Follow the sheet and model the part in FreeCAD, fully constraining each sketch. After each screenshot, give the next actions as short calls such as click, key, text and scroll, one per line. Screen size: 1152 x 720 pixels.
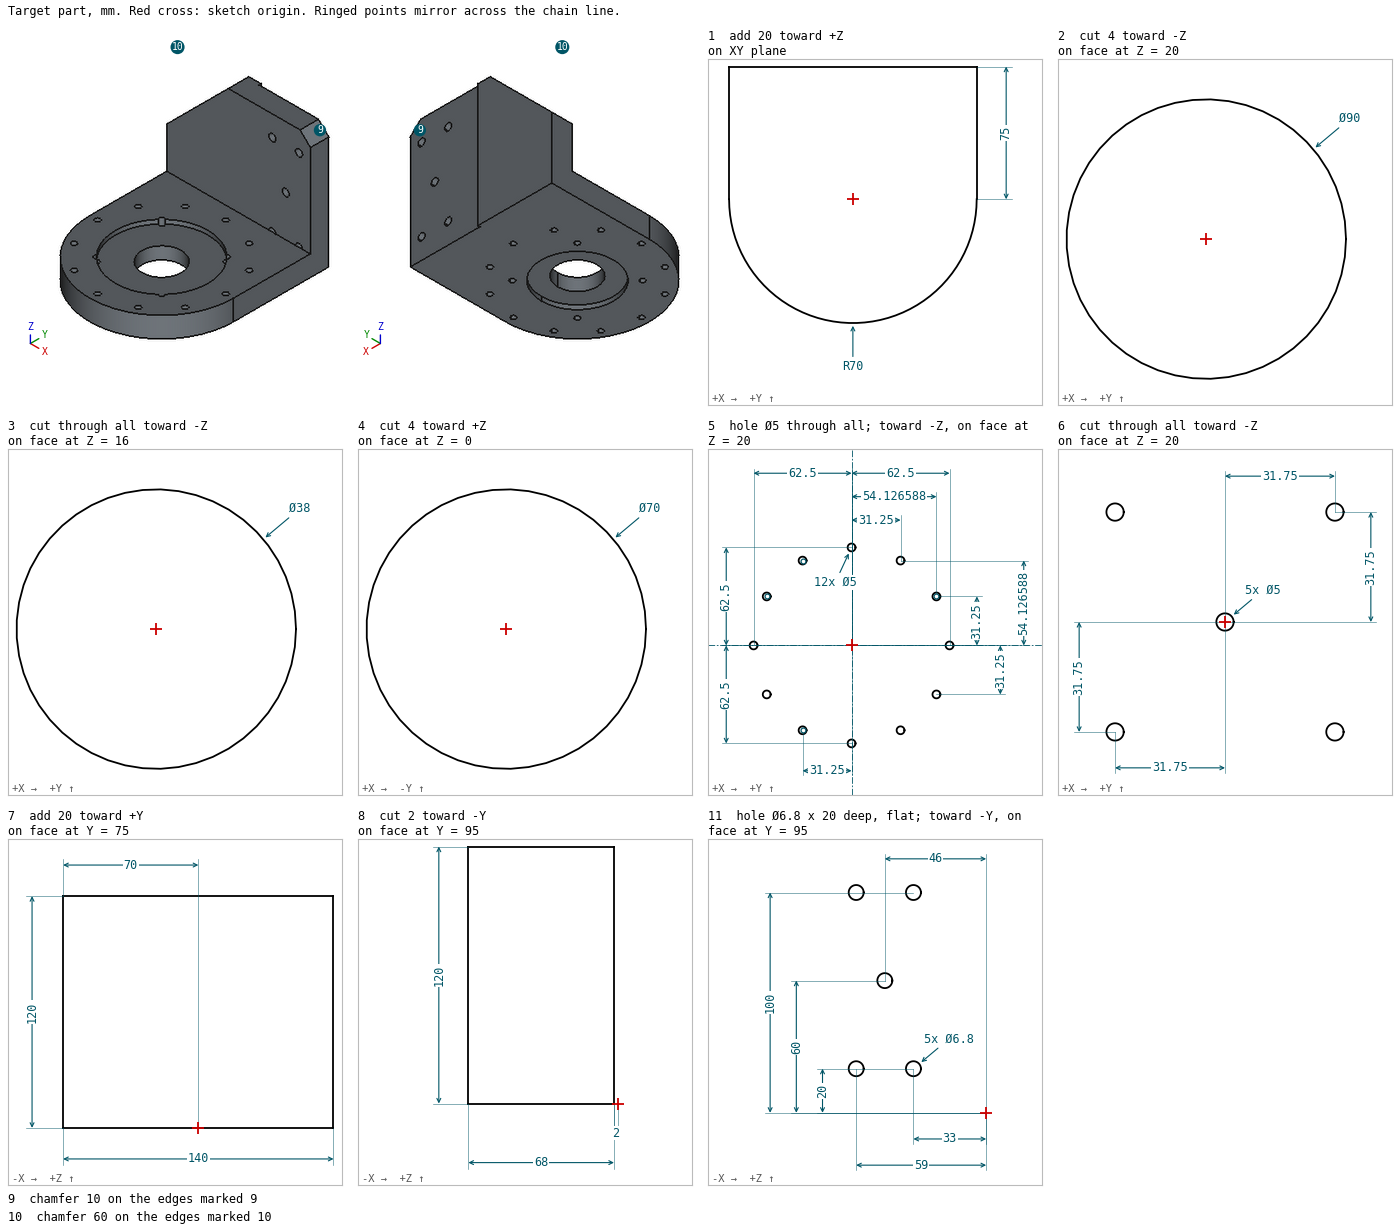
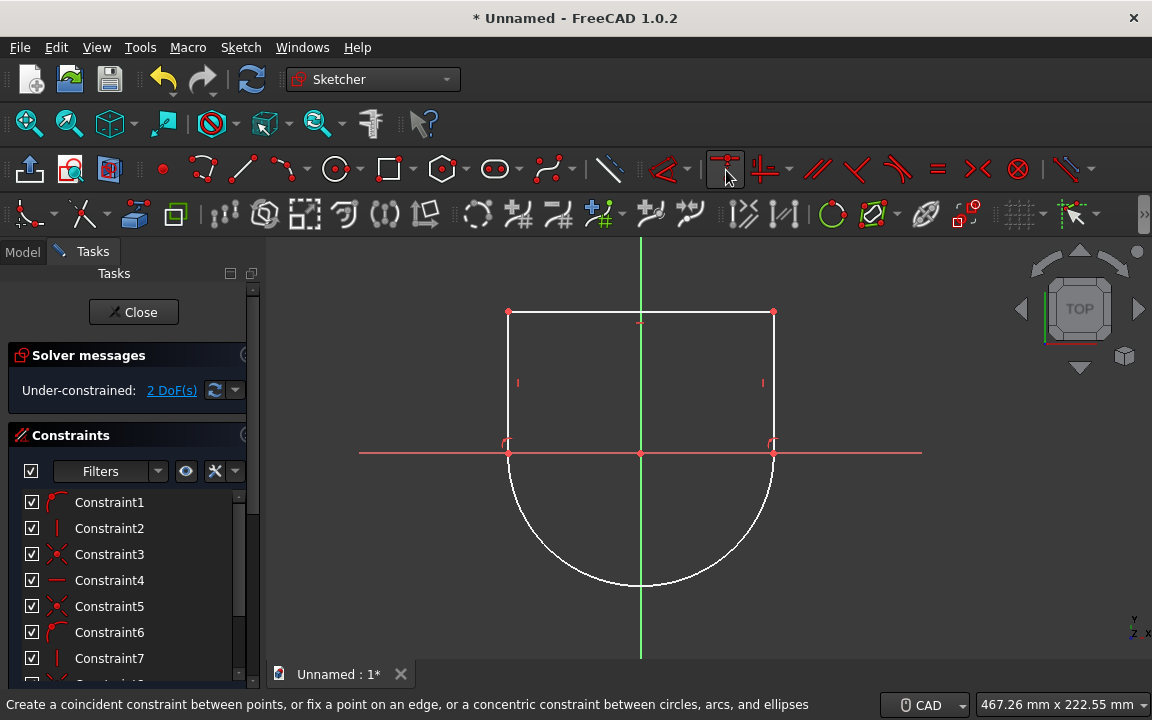
click(664, 170)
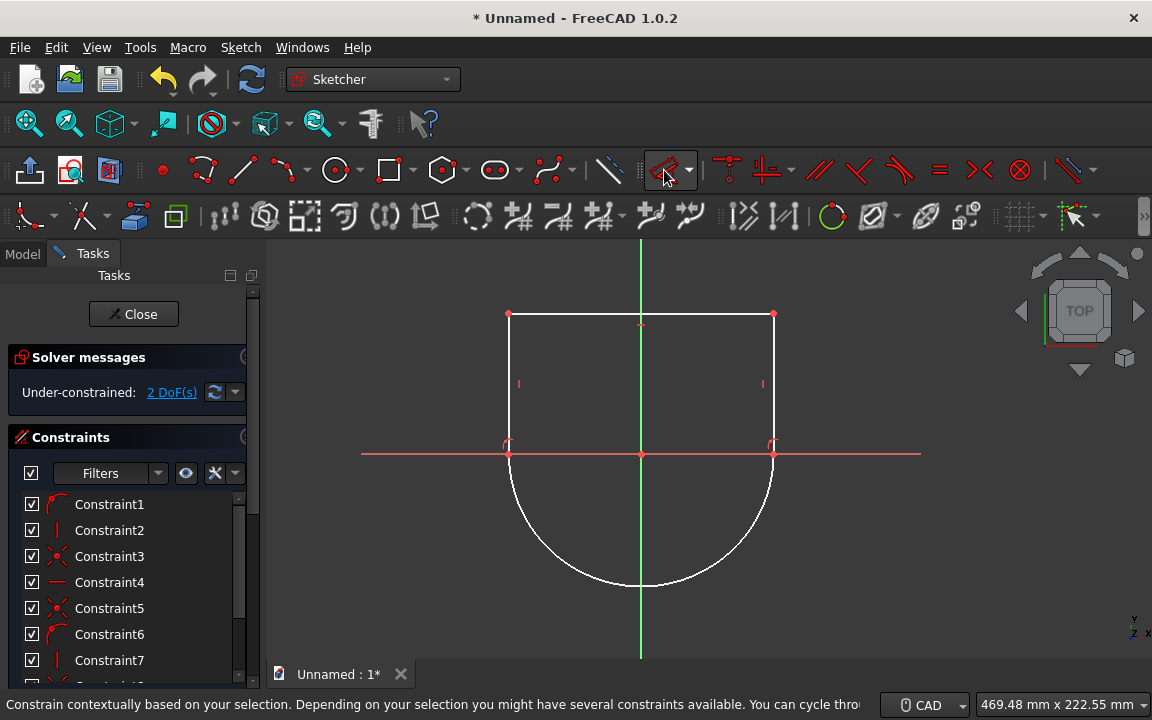
click(563, 561)
click(544, 587)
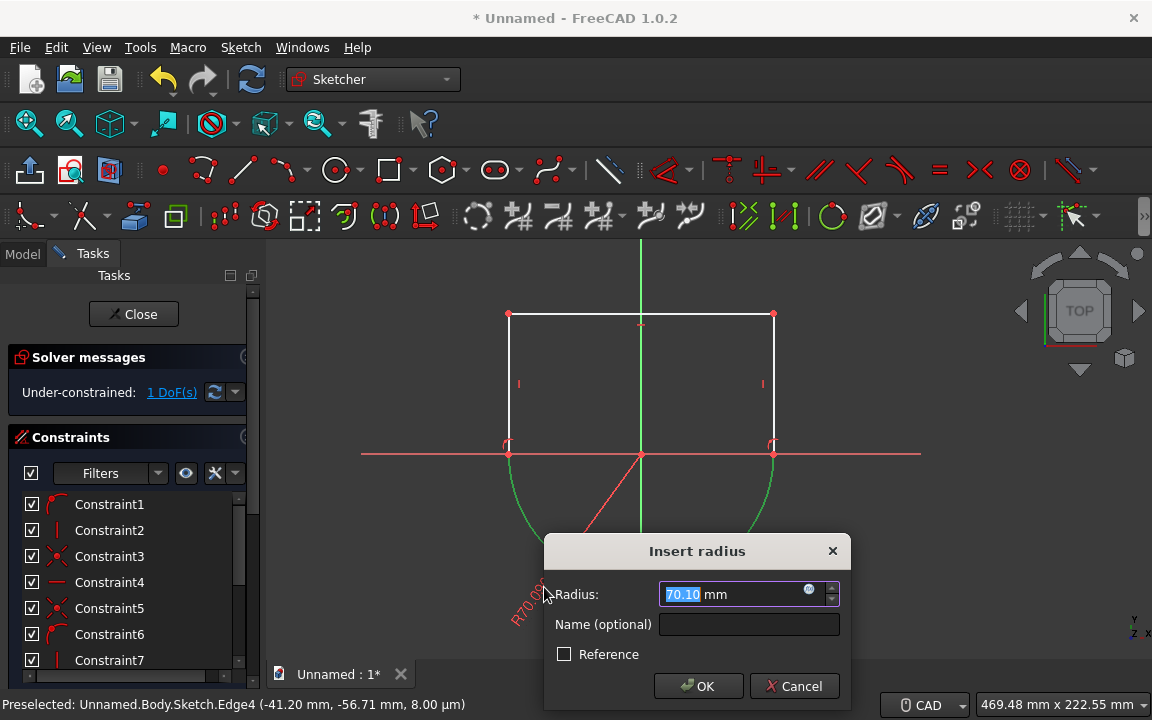
text(70)
key(Return)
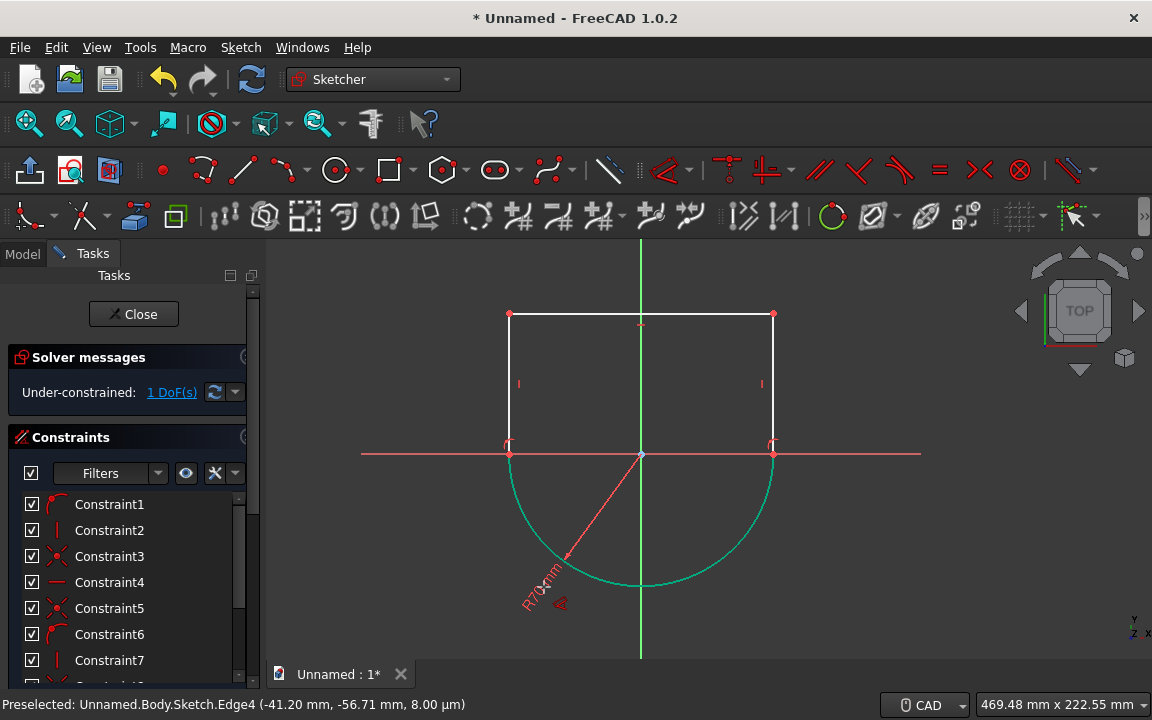
click(773, 412)
click(807, 384)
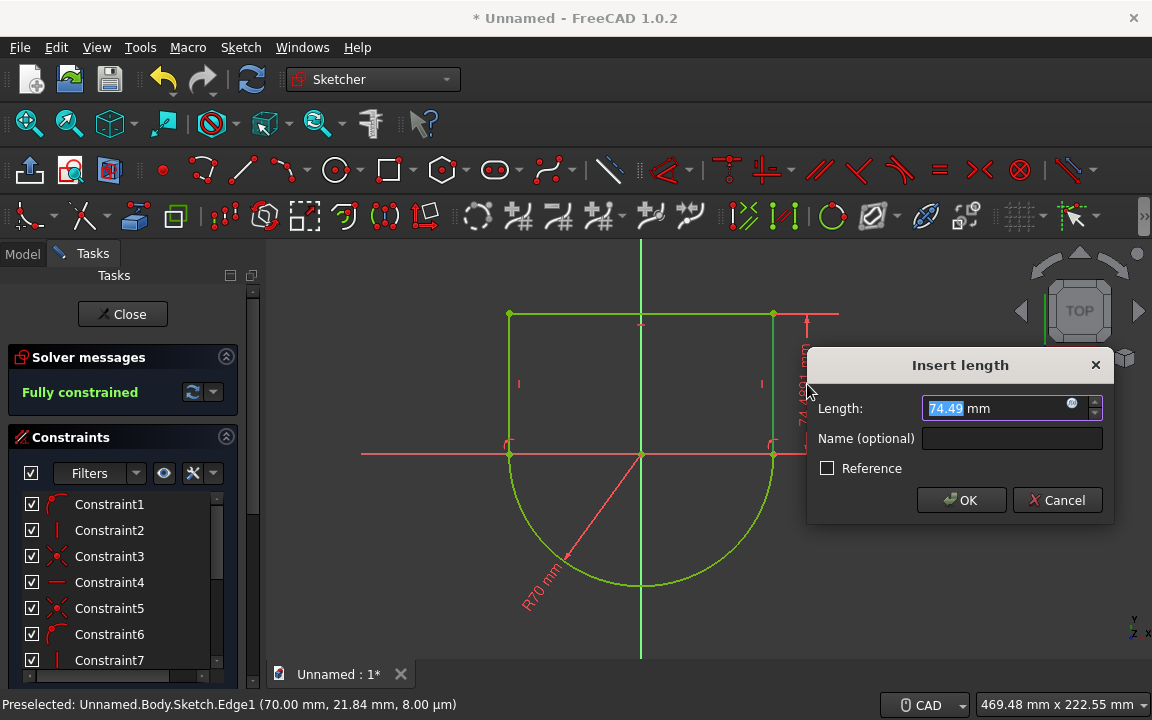
text(75)
key(Return)
key(Escape)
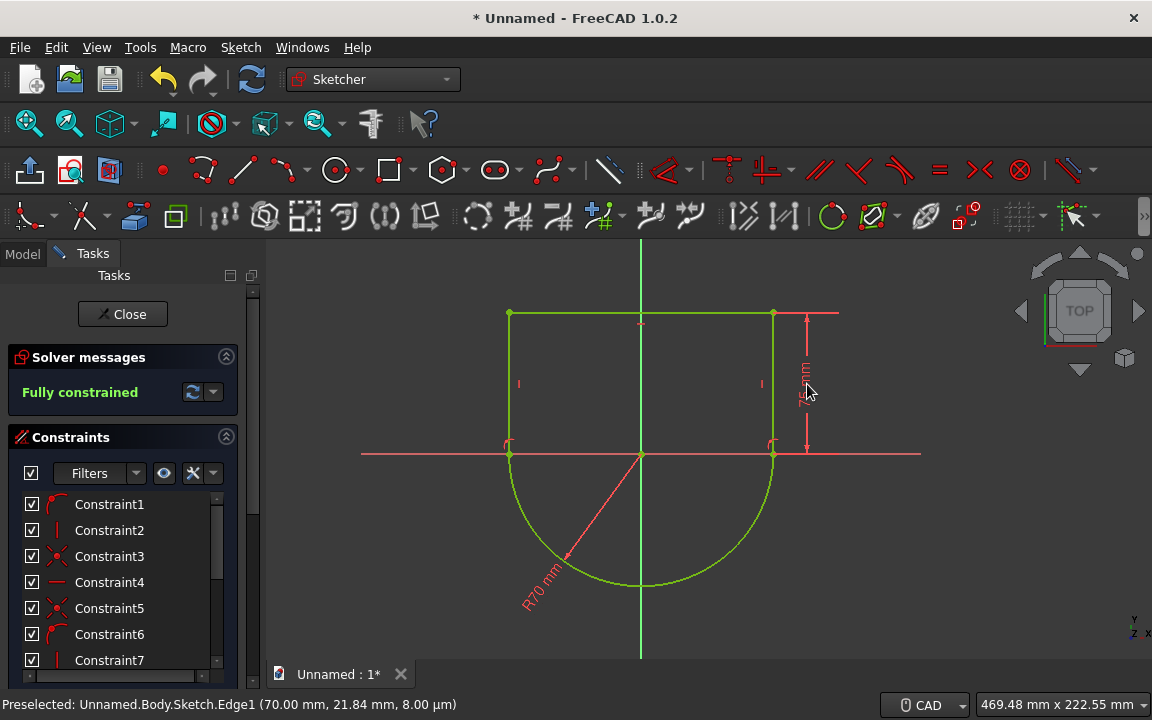
click(123, 314)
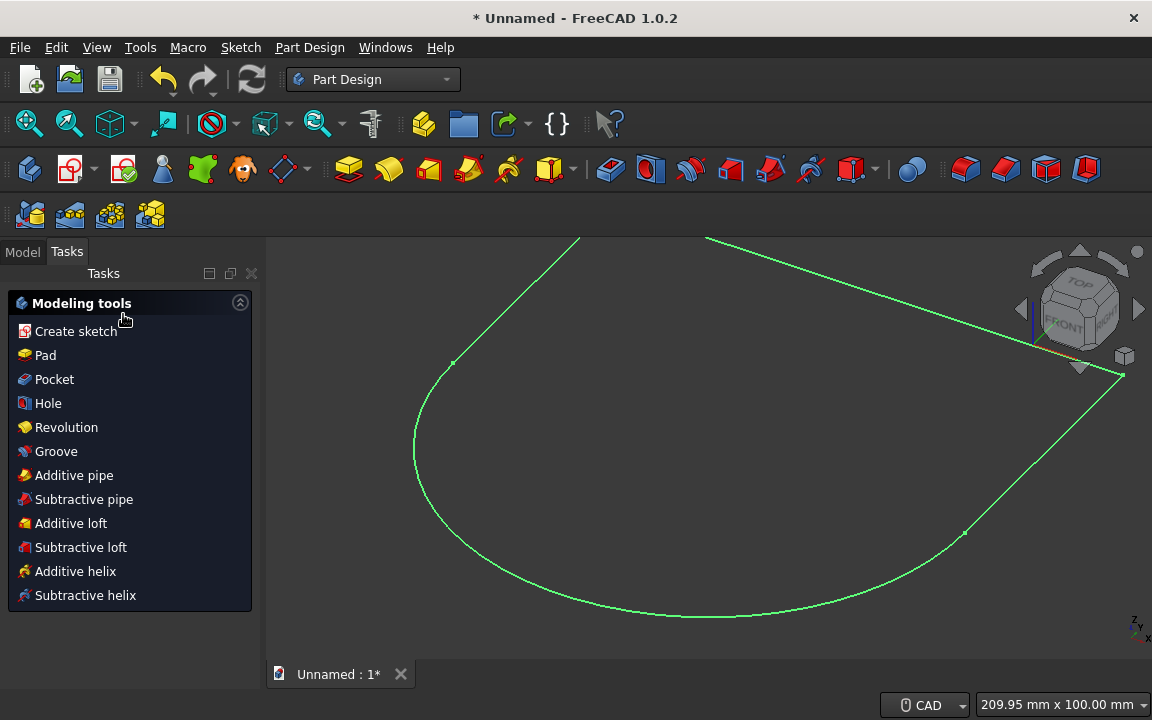
click(350, 170)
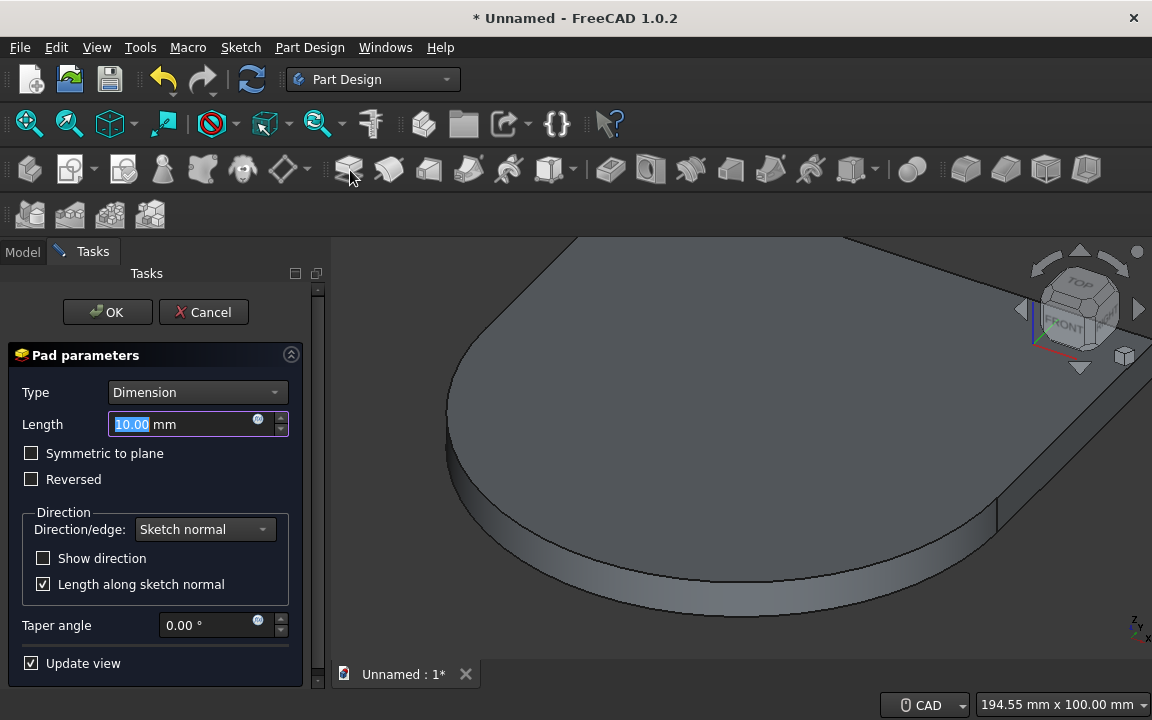
text(20)
key(Tab)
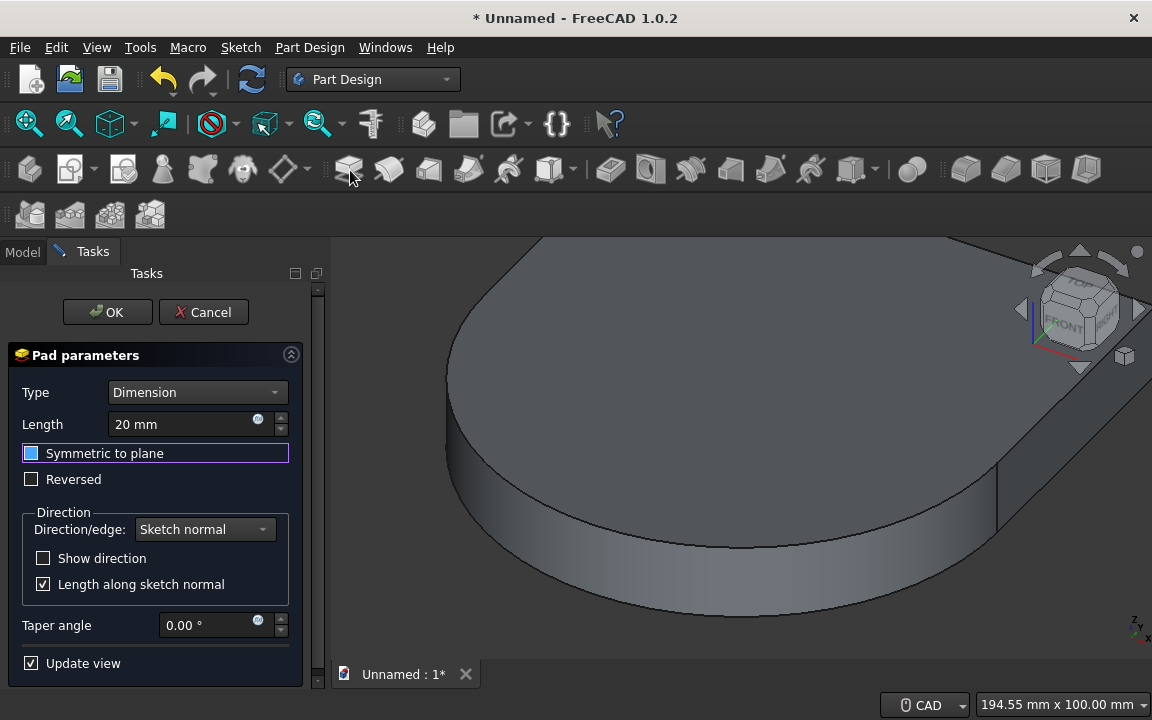
click(108, 312)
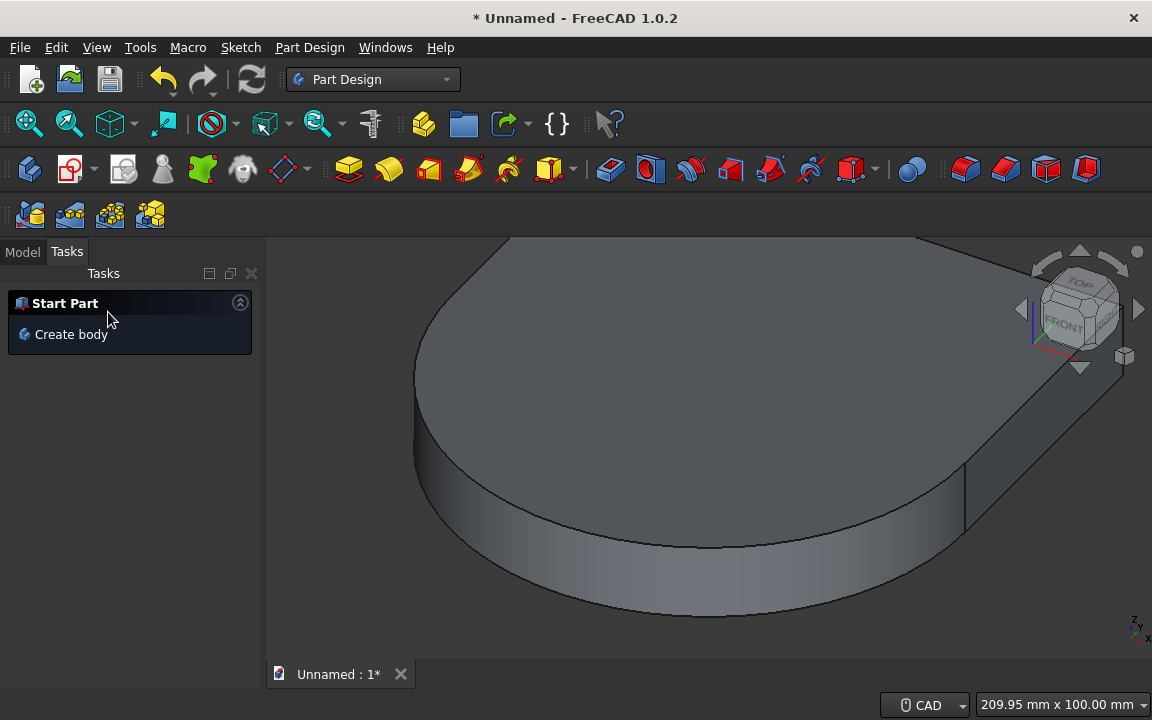
click(30, 124)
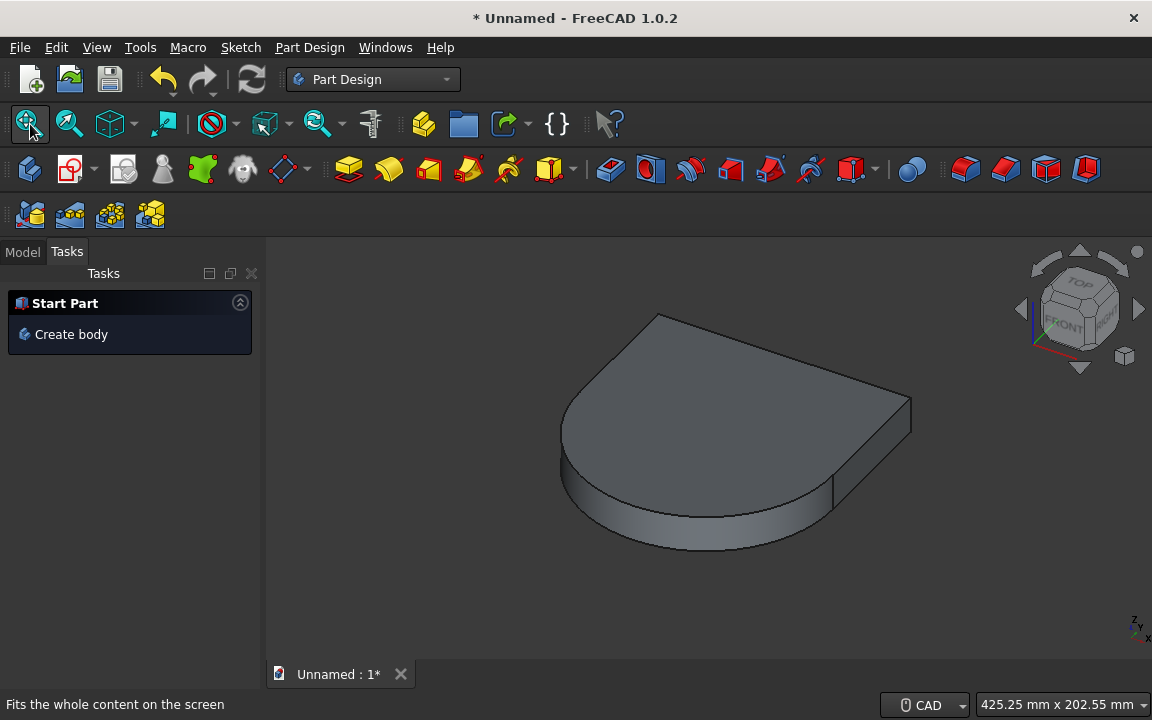
click(709, 430)